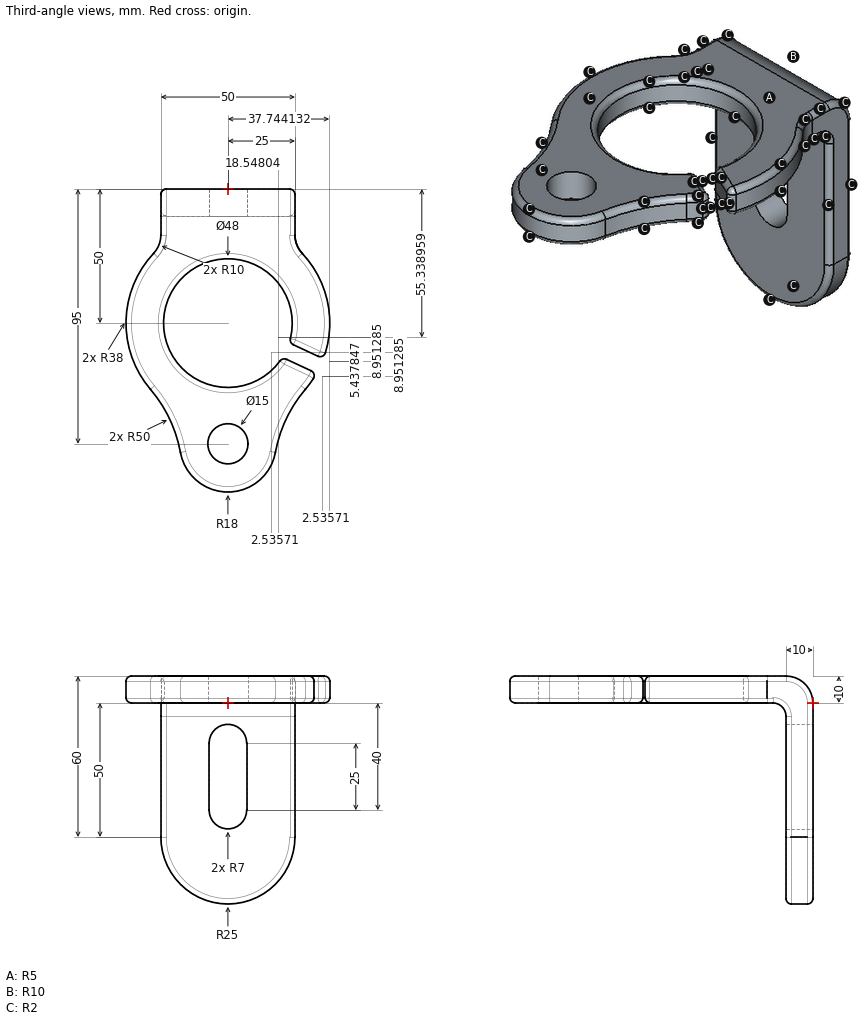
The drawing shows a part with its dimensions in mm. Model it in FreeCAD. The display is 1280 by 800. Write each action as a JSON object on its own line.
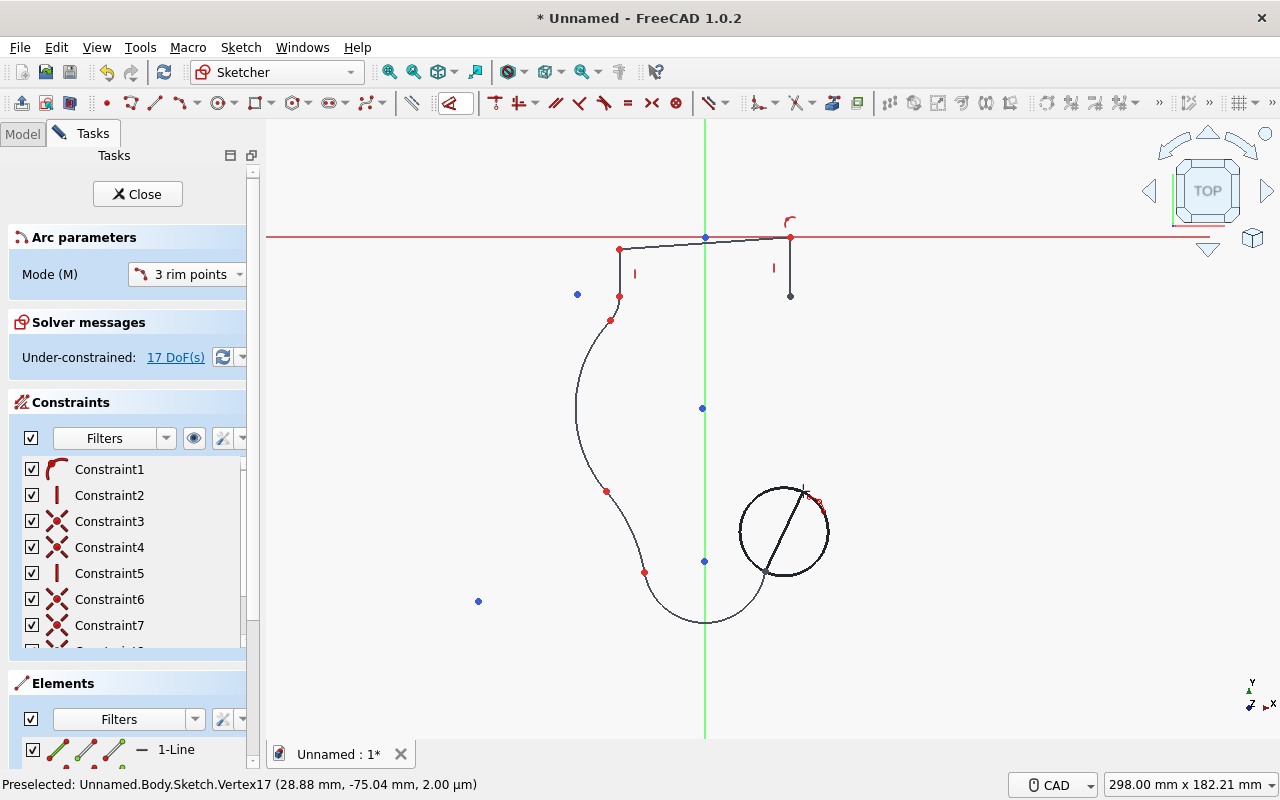
{"action": "scroll", "coordinate": [779, 529], "scroll_direction": "up", "scroll_amount": 5}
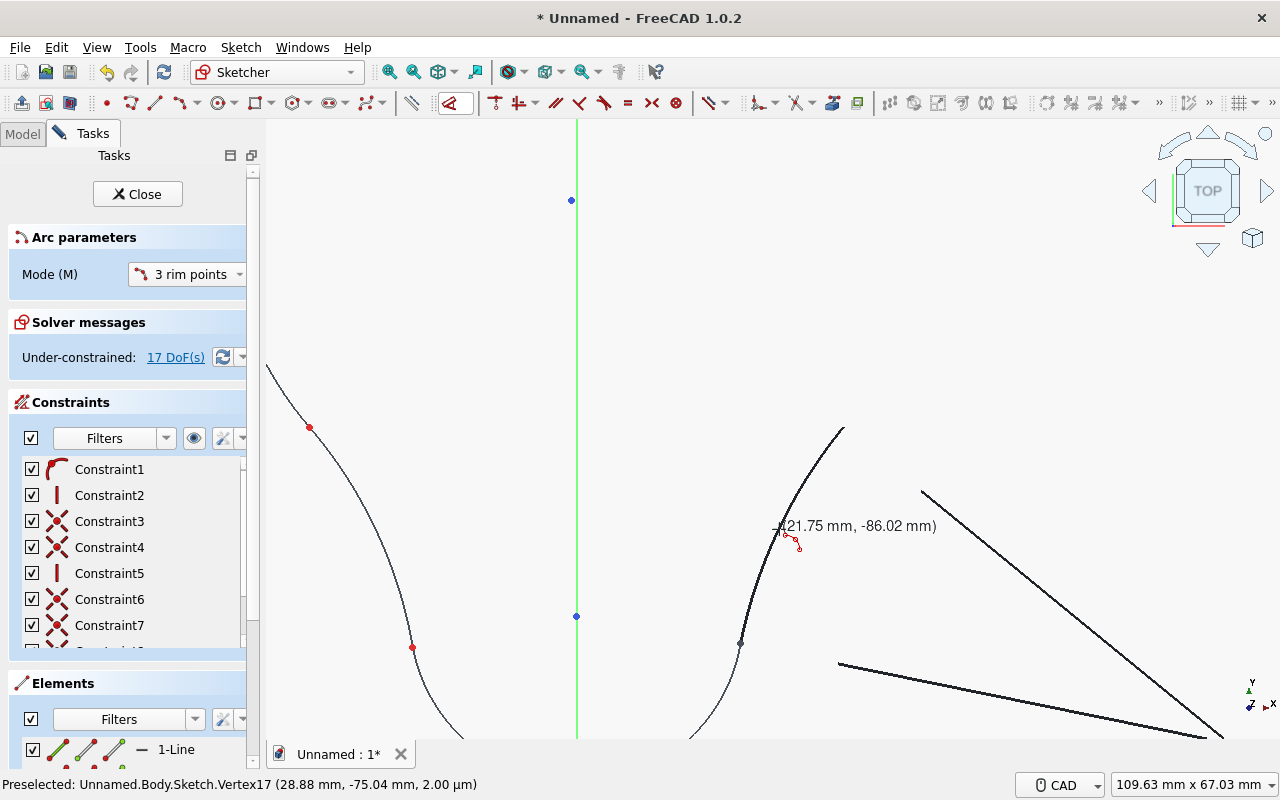
{"action": "left_click", "coordinate": [778, 528]}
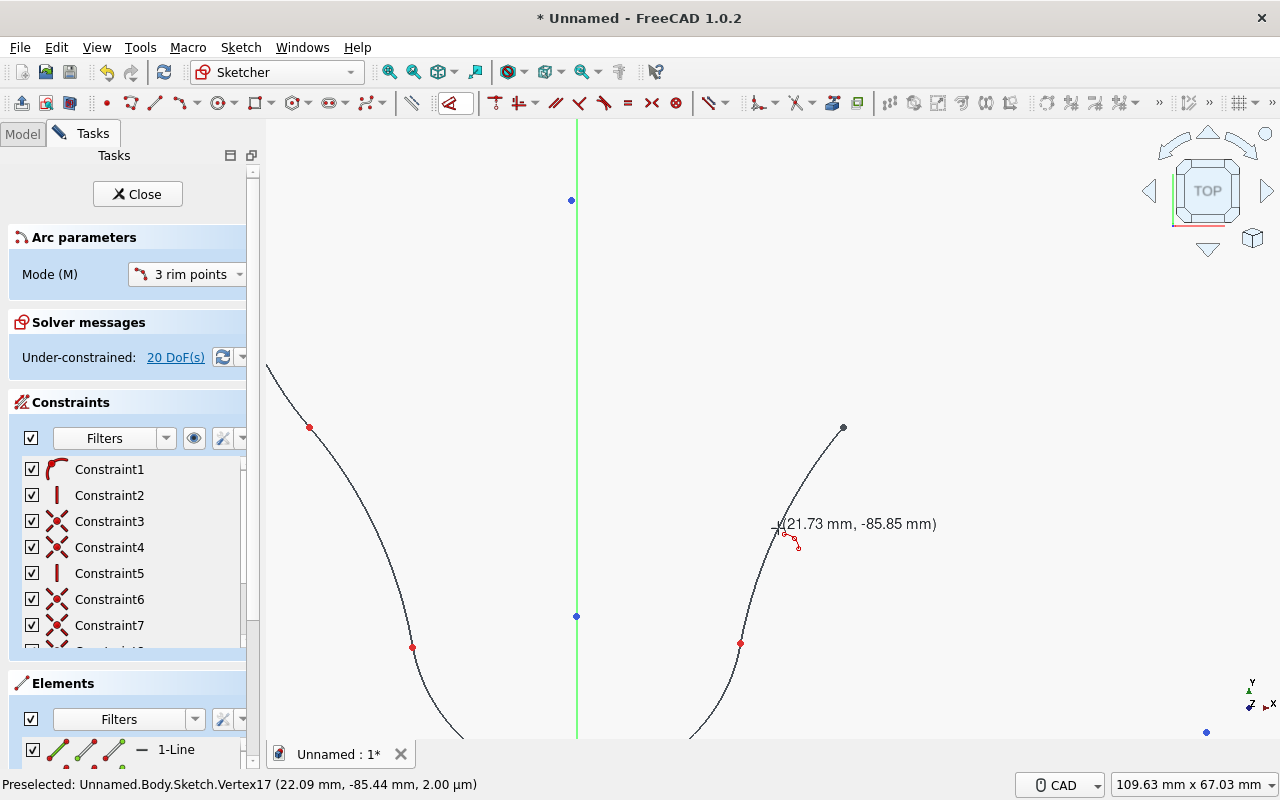
{"action": "left_click", "coordinate": [843, 427]}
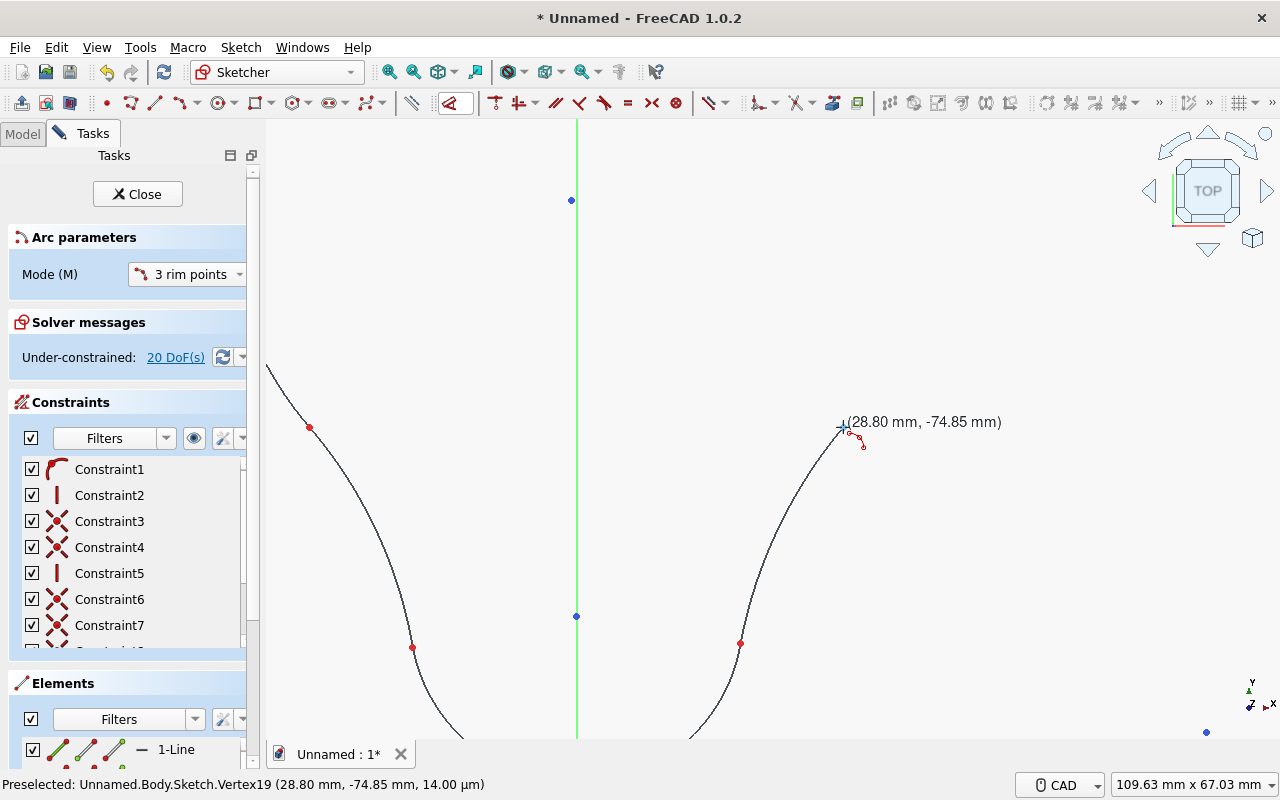
{"action": "scroll", "coordinate": [779, 529], "scroll_direction": "down", "scroll_amount": 5}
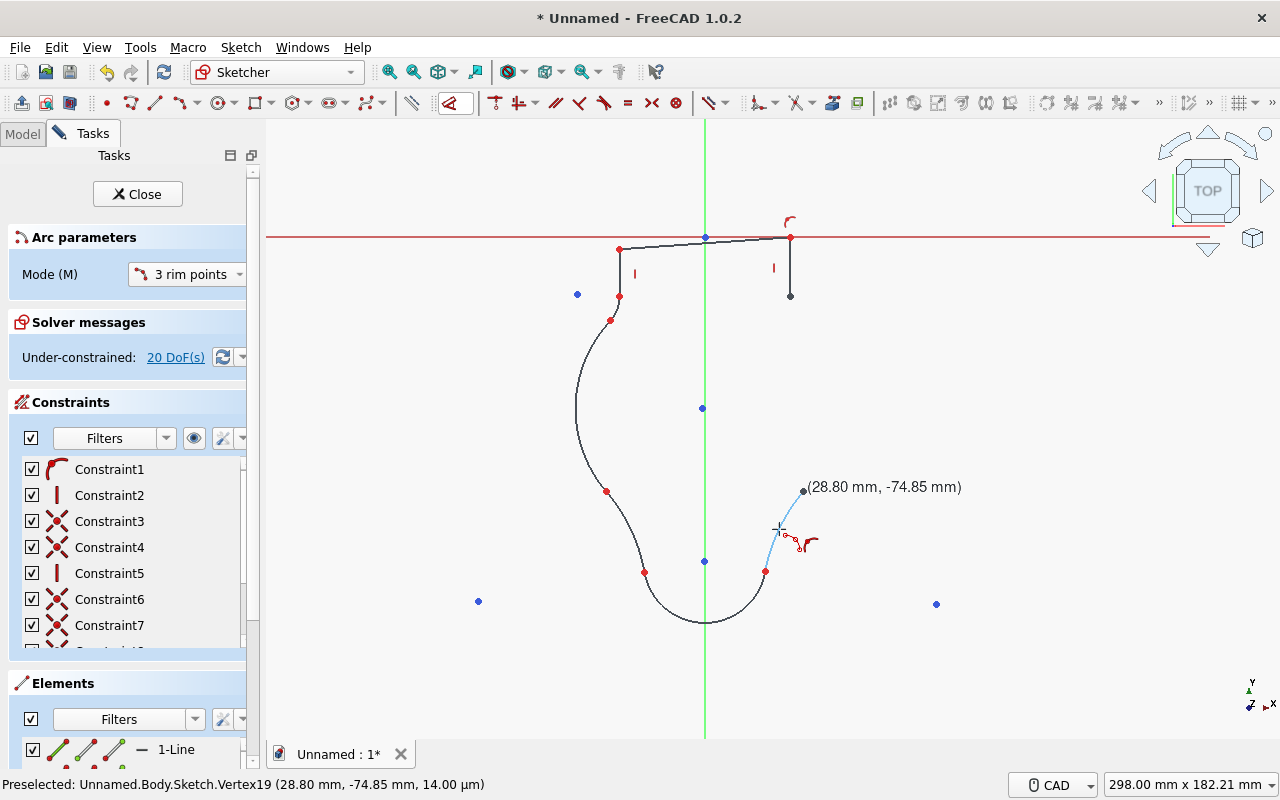
{"action": "left_click", "coordinate": [799, 319]}
{"action": "left_click", "coordinate": [834, 404]}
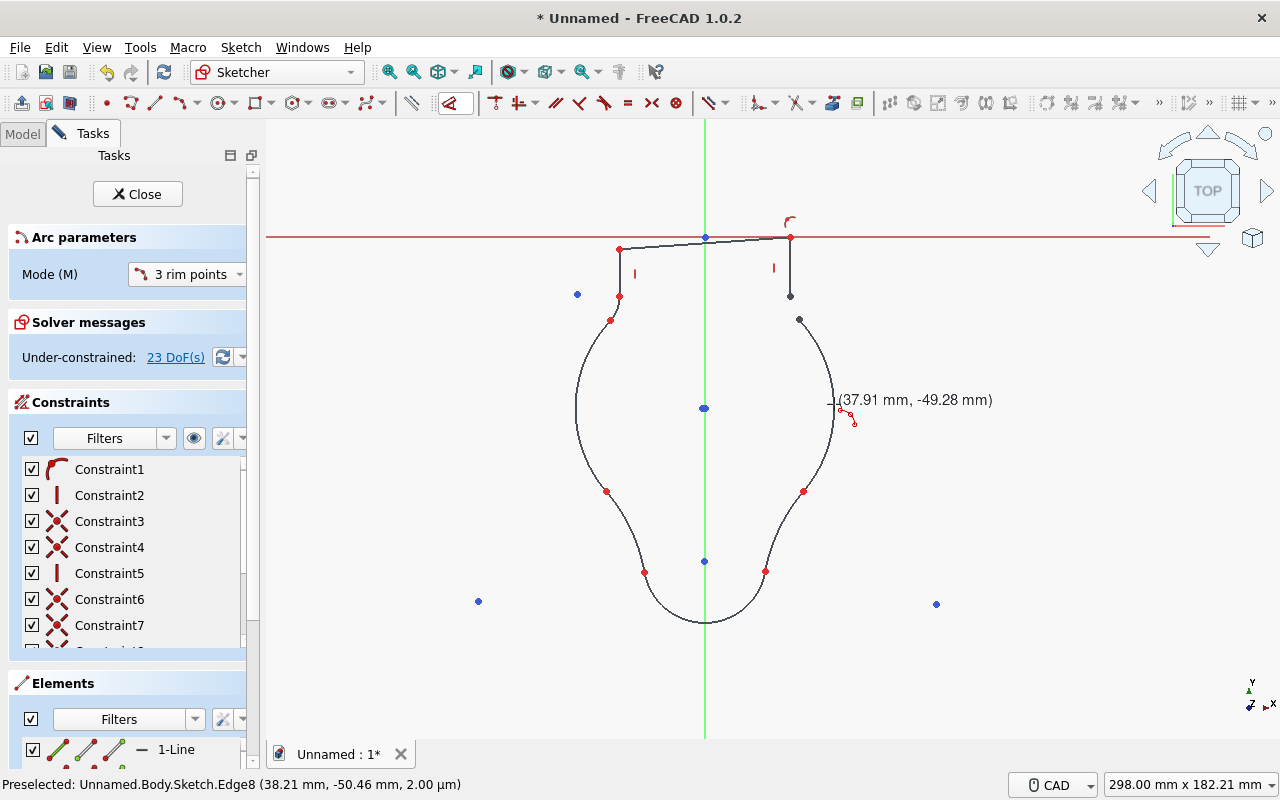
{"action": "left_click", "coordinate": [799, 320]}
{"action": "left_click", "coordinate": [790, 297]}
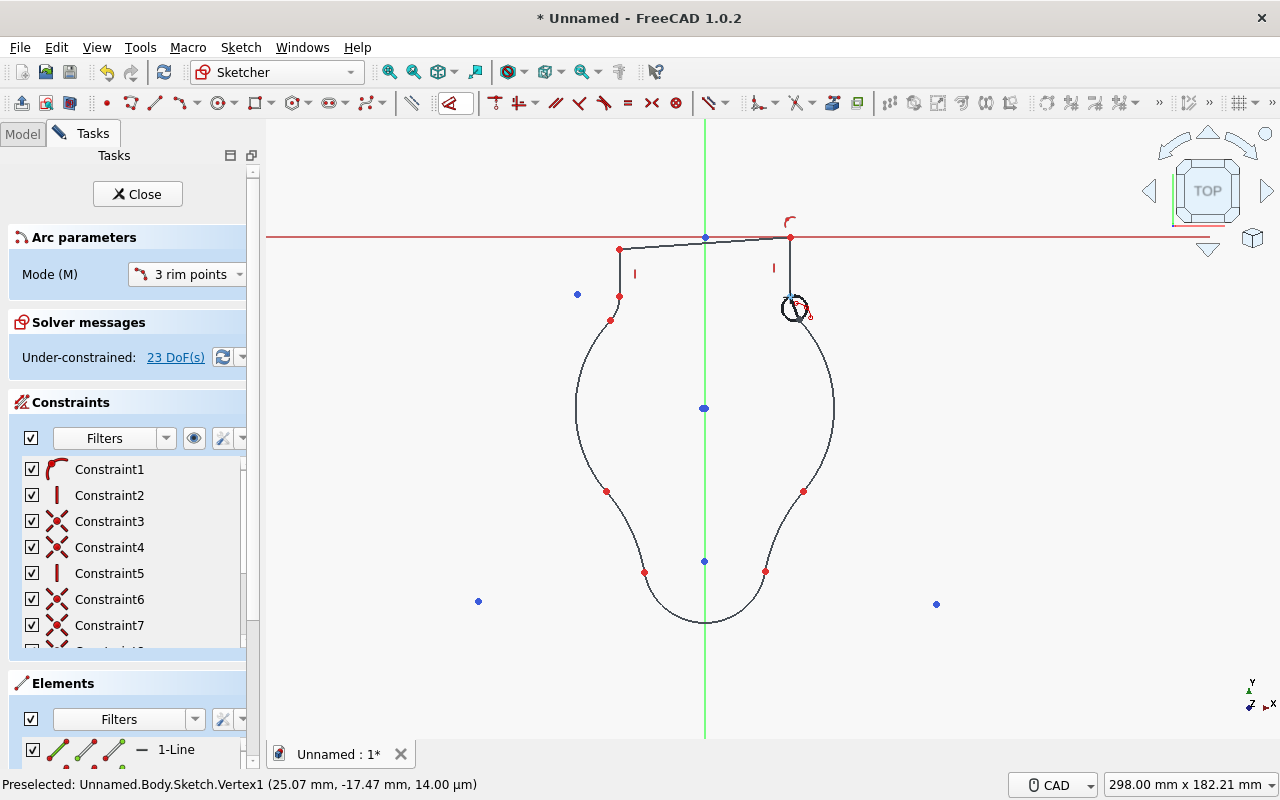
{"action": "scroll", "coordinate": [792, 308], "scroll_direction": "up", "scroll_amount": 10}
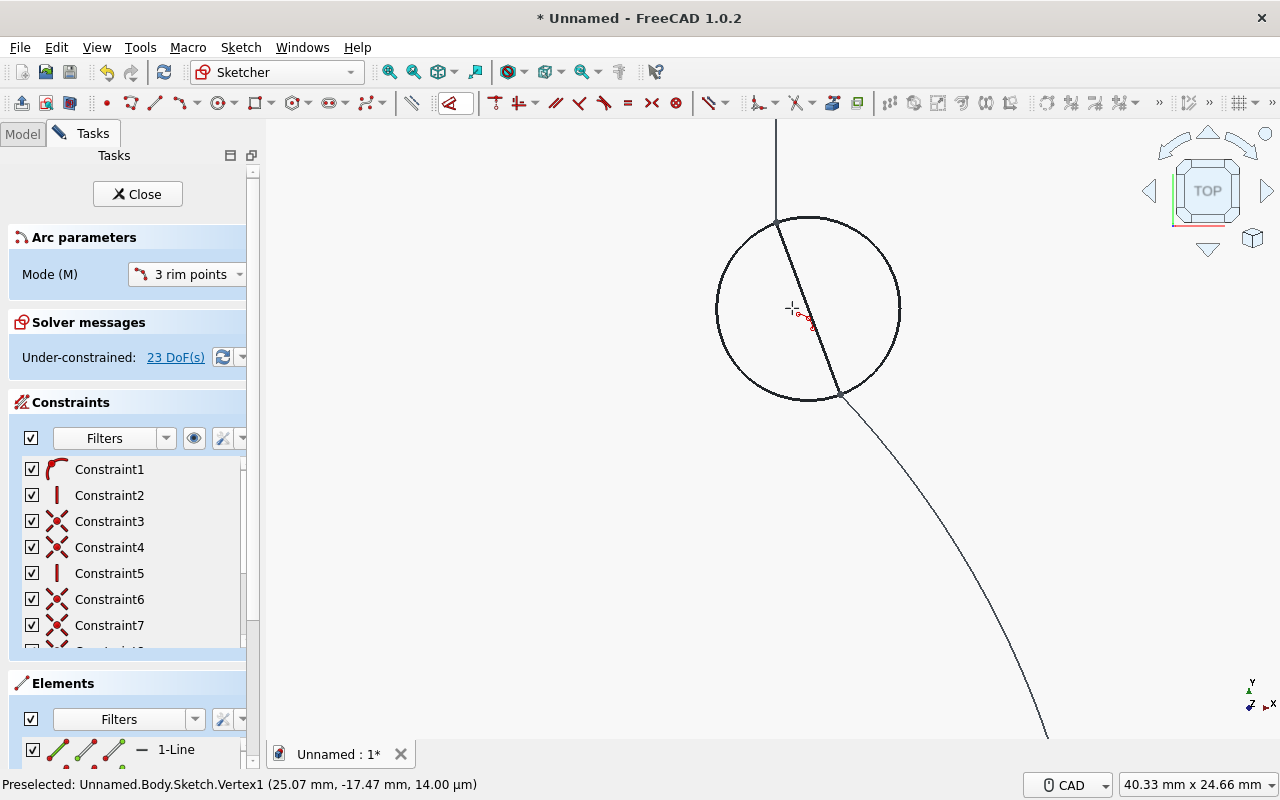
{"action": "left_click", "coordinate": [792, 308]}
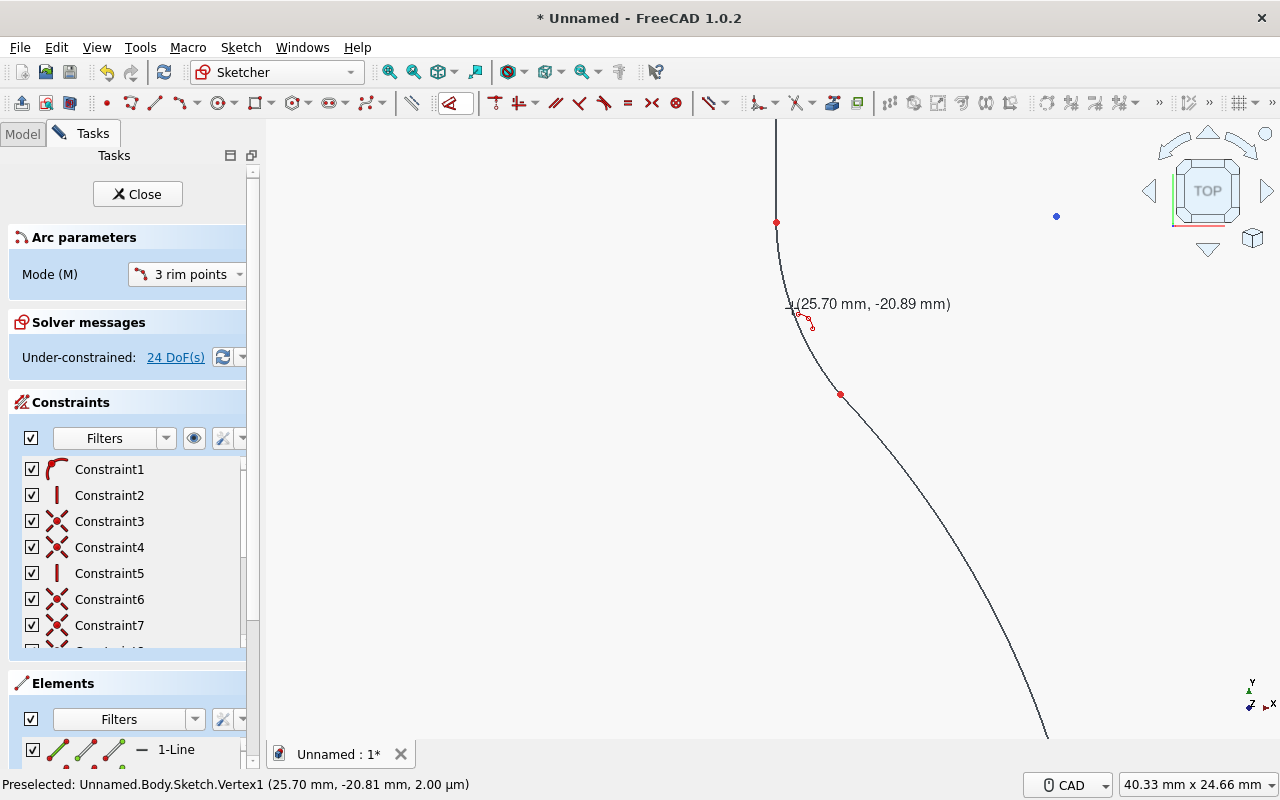
{"action": "left_click", "coordinate": [218, 104]}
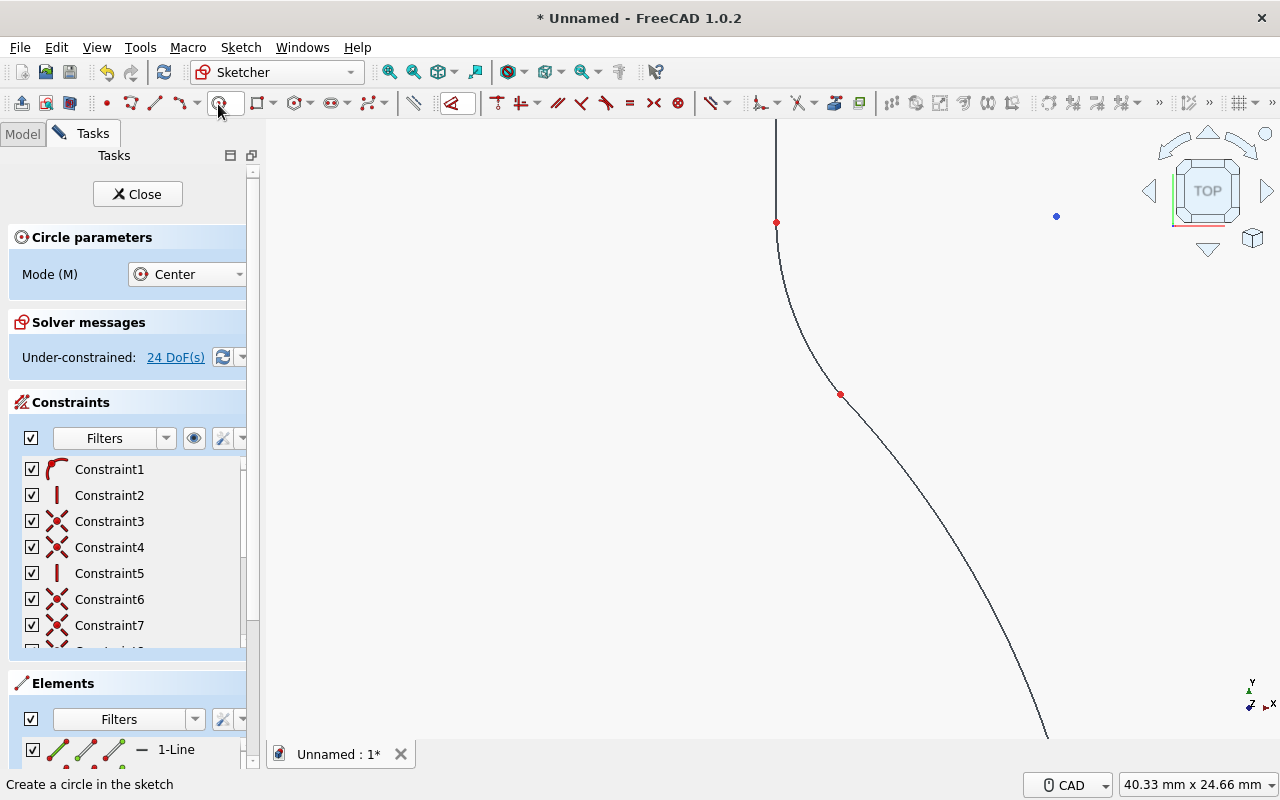
{"action": "scroll", "coordinate": [792, 308], "scroll_direction": "down", "scroll_amount": 10}